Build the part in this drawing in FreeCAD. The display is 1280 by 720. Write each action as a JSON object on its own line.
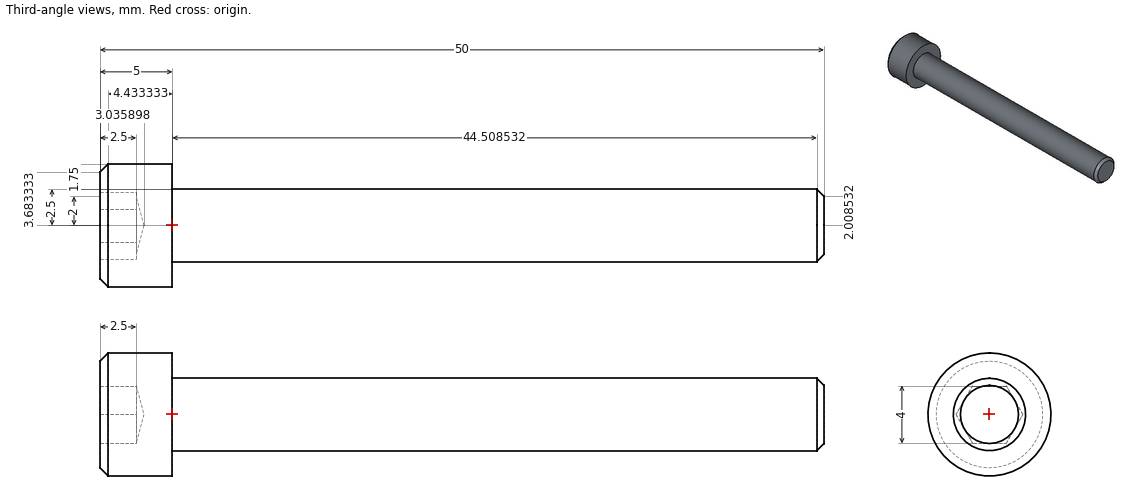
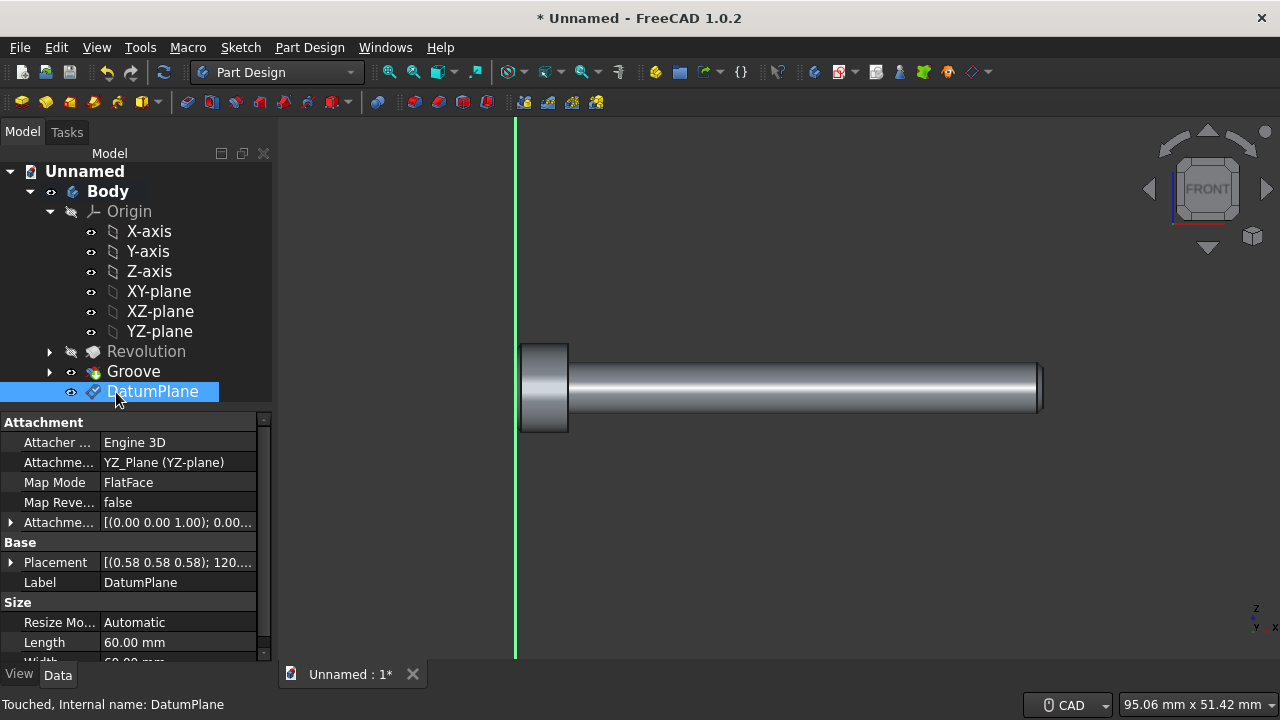
{"action": "left_click", "coordinate": [840, 72]}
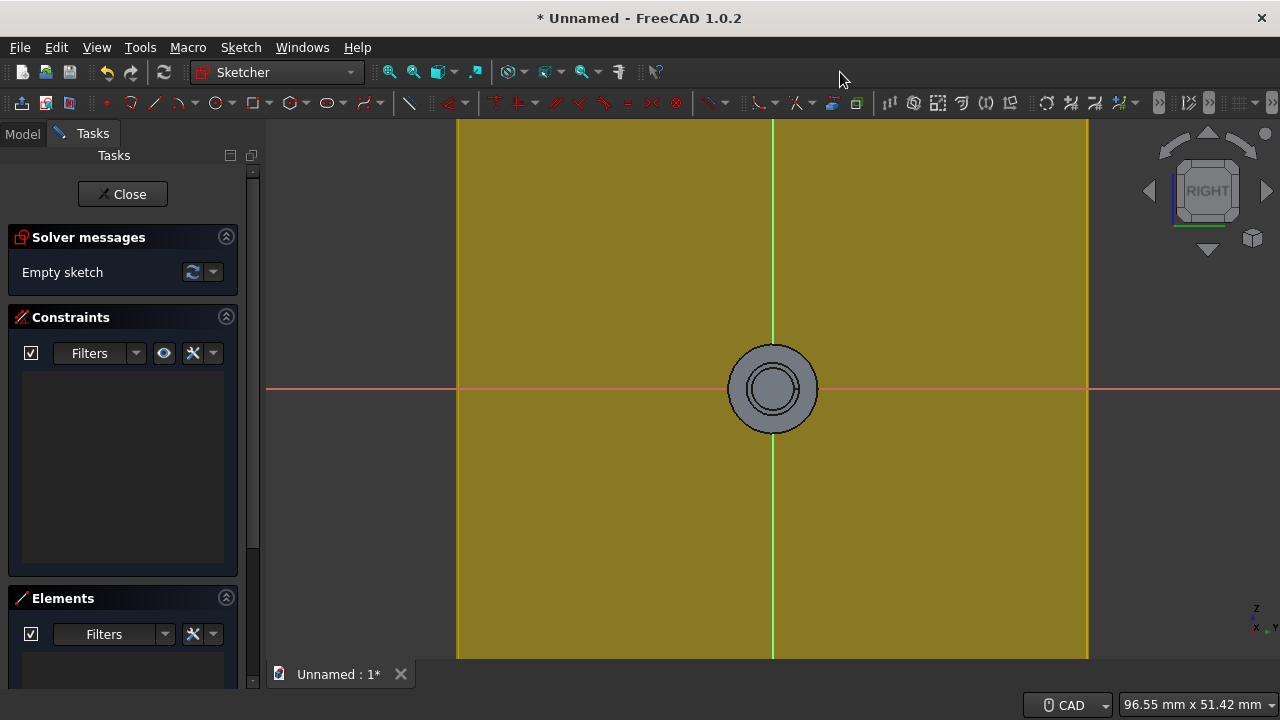
{"action": "key", "text": "q s"}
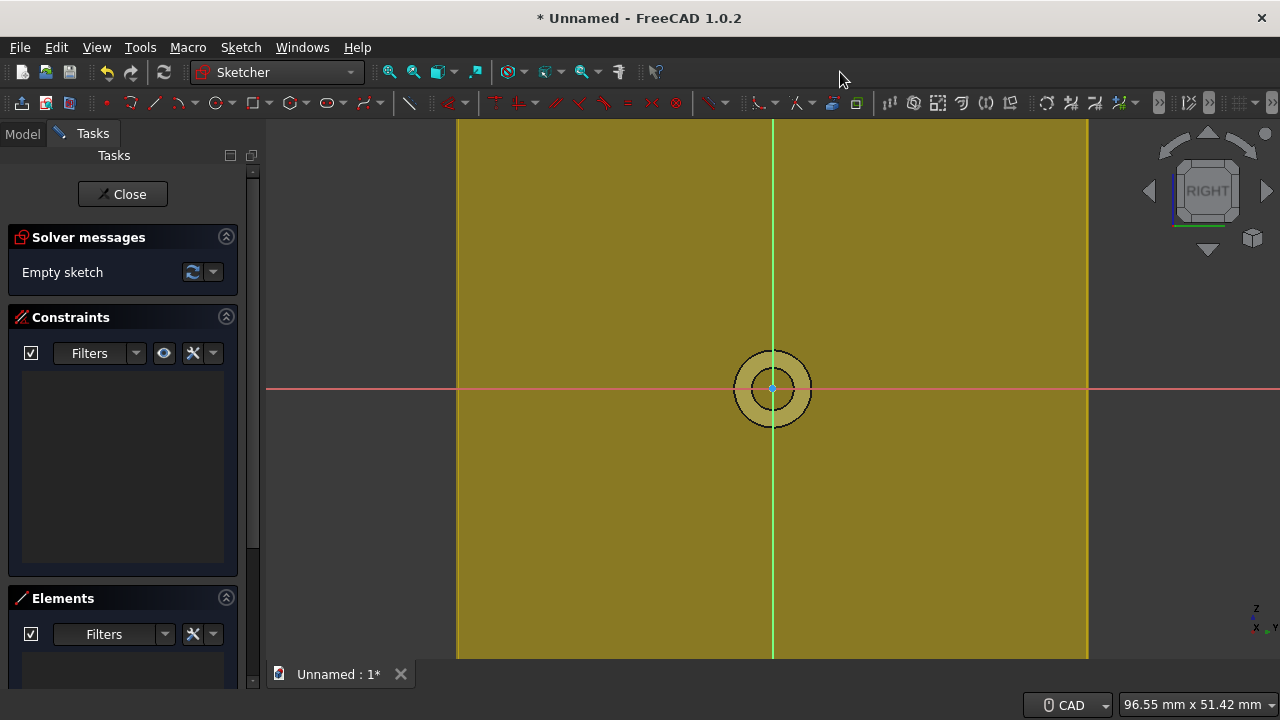
{"action": "scroll", "coordinate": [784, 389], "scroll_direction": "up", "scroll_amount": 10}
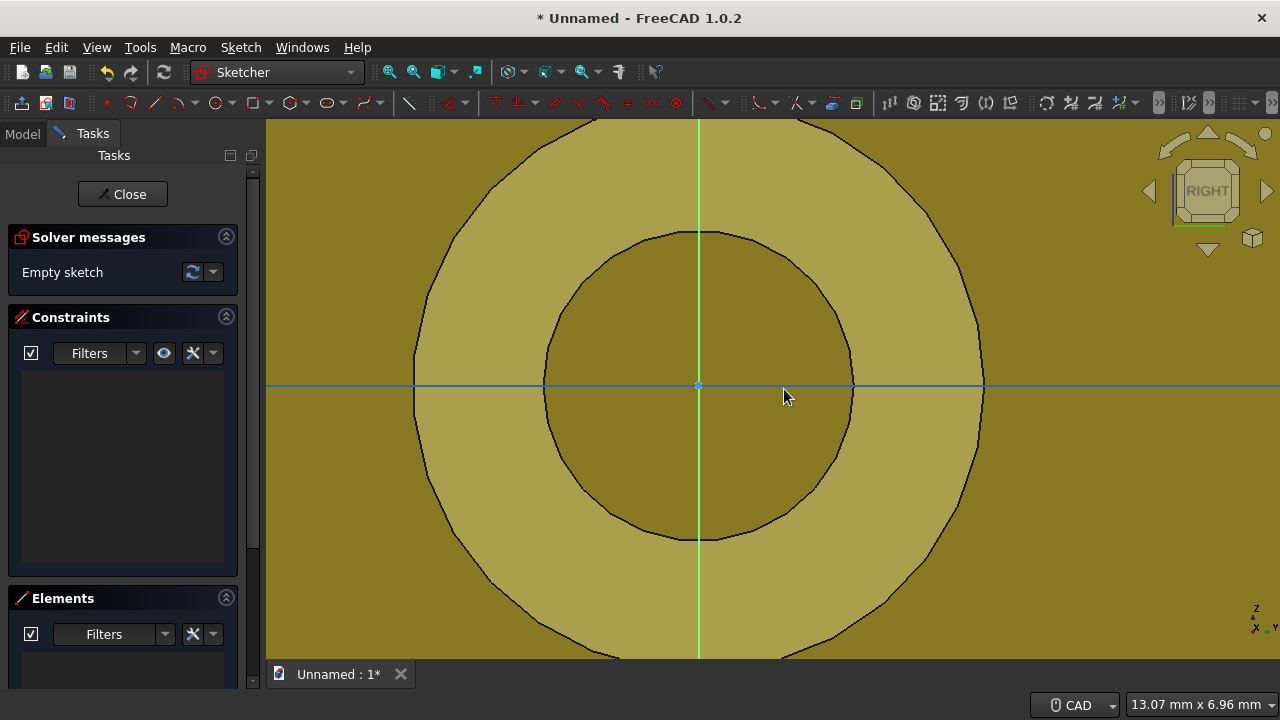
{"action": "left_click", "coordinate": [290, 104]}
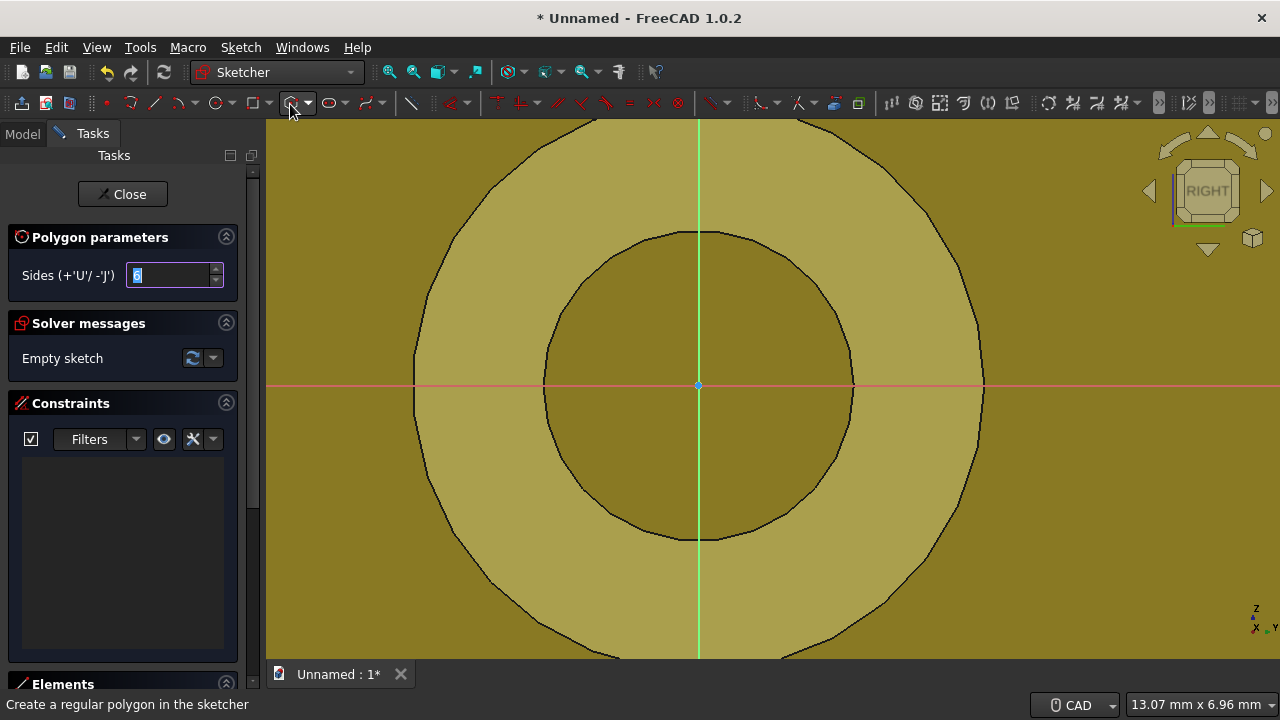
{"action": "left_click", "coordinate": [699, 386]}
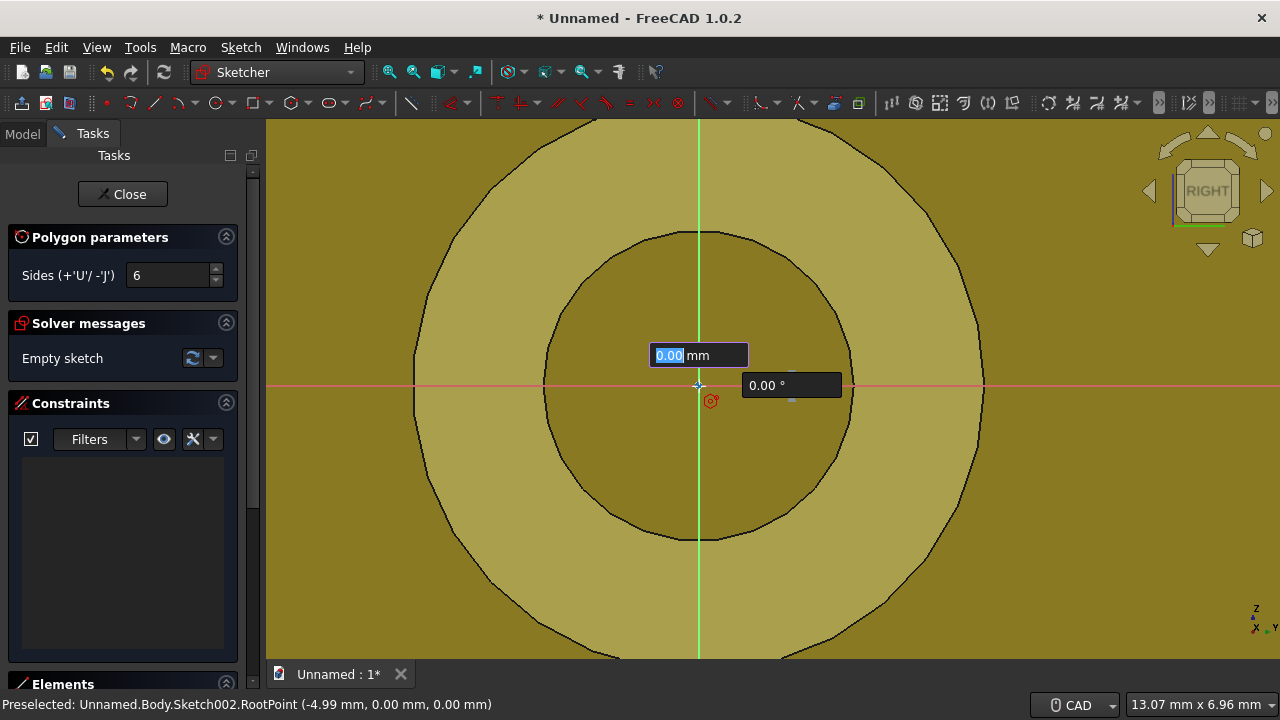
{"action": "left_click", "coordinate": [519, 386]}
{"action": "right_click", "coordinate": [519, 386]}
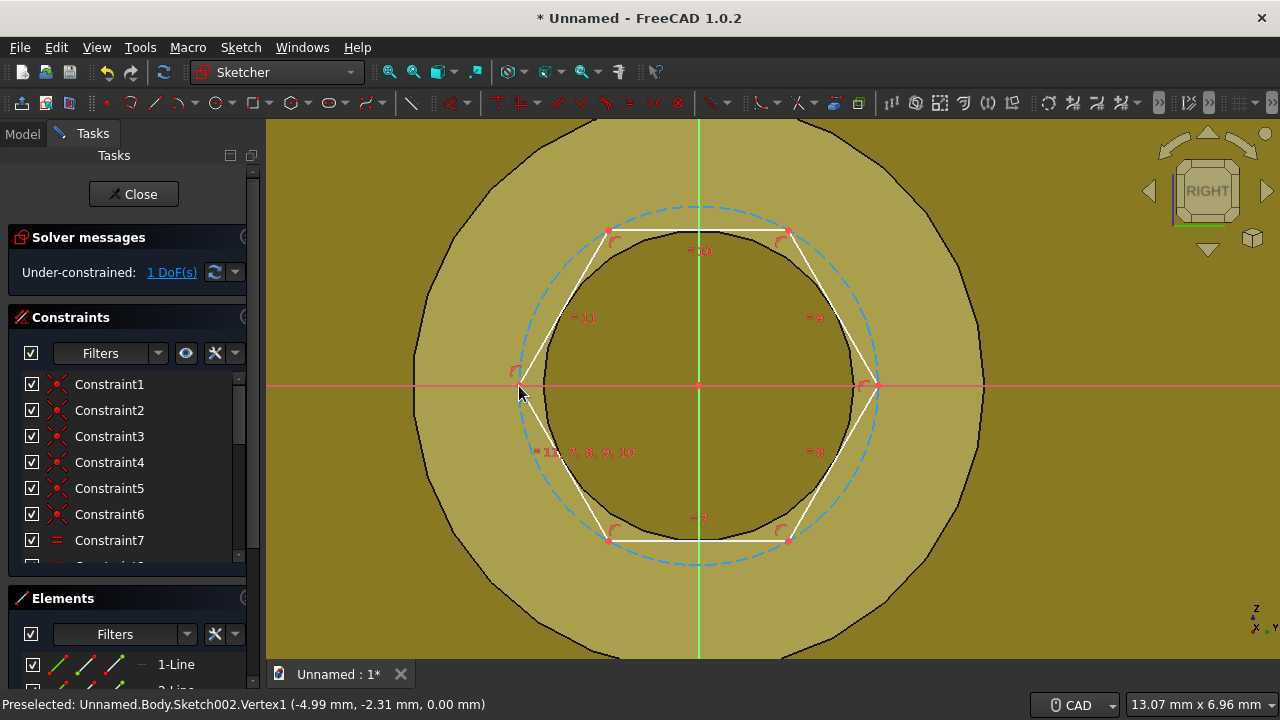
{"action": "key", "text": "d"}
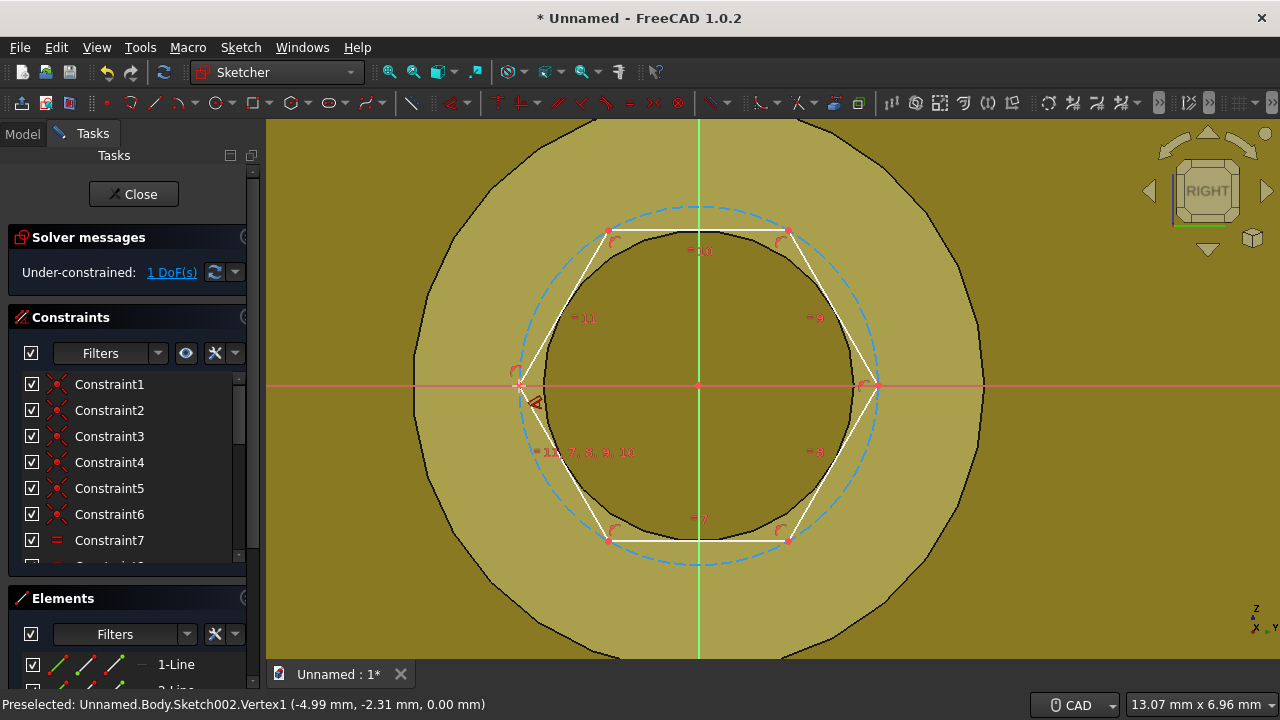
{"action": "left_click", "coordinate": [609, 541]}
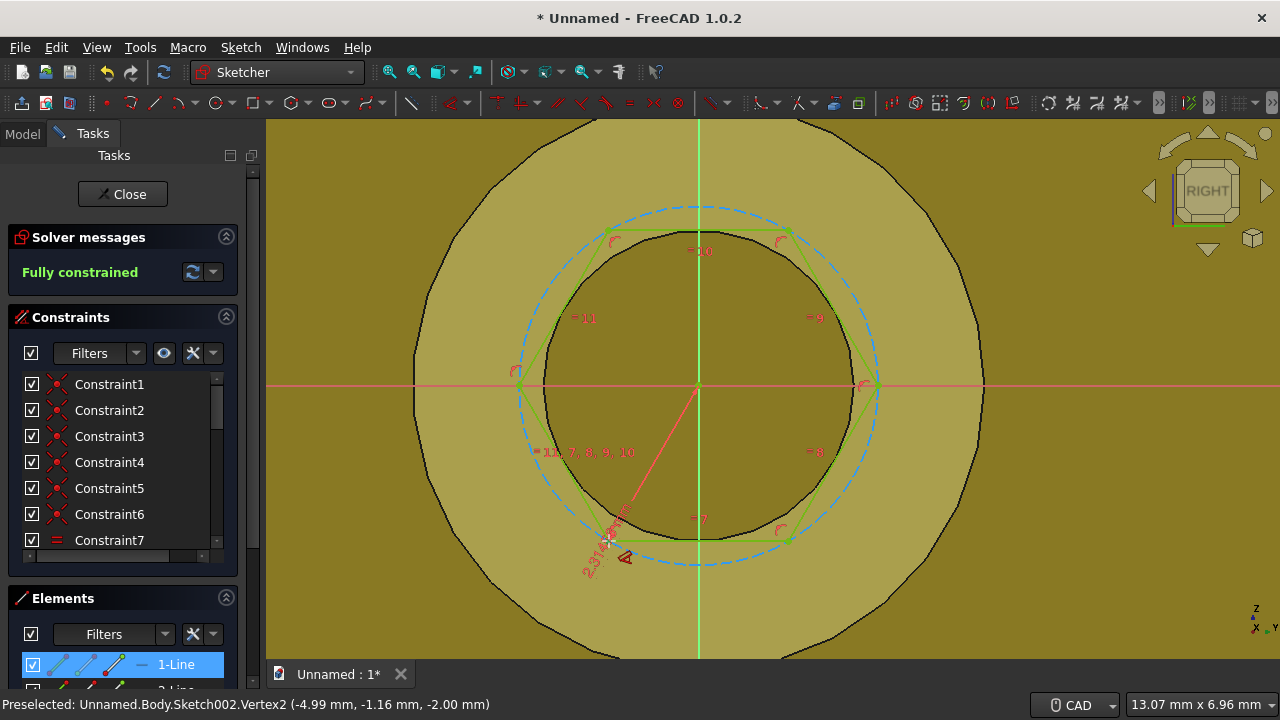
{"action": "left_click", "coordinate": [788, 230]}
{"action": "left_click", "coordinate": [870, 277]}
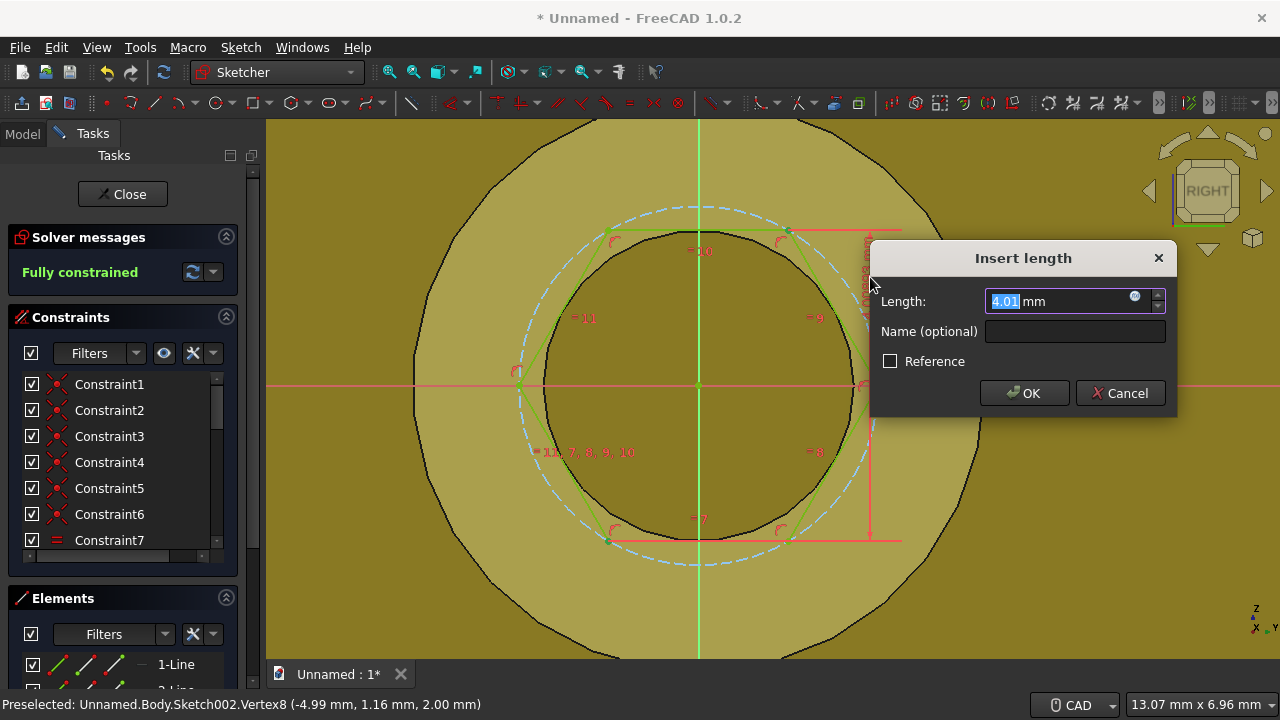
{"action": "type", "text": "4"}
{"action": "key", "text": "Return"}
{"action": "key", "text": "Escape"}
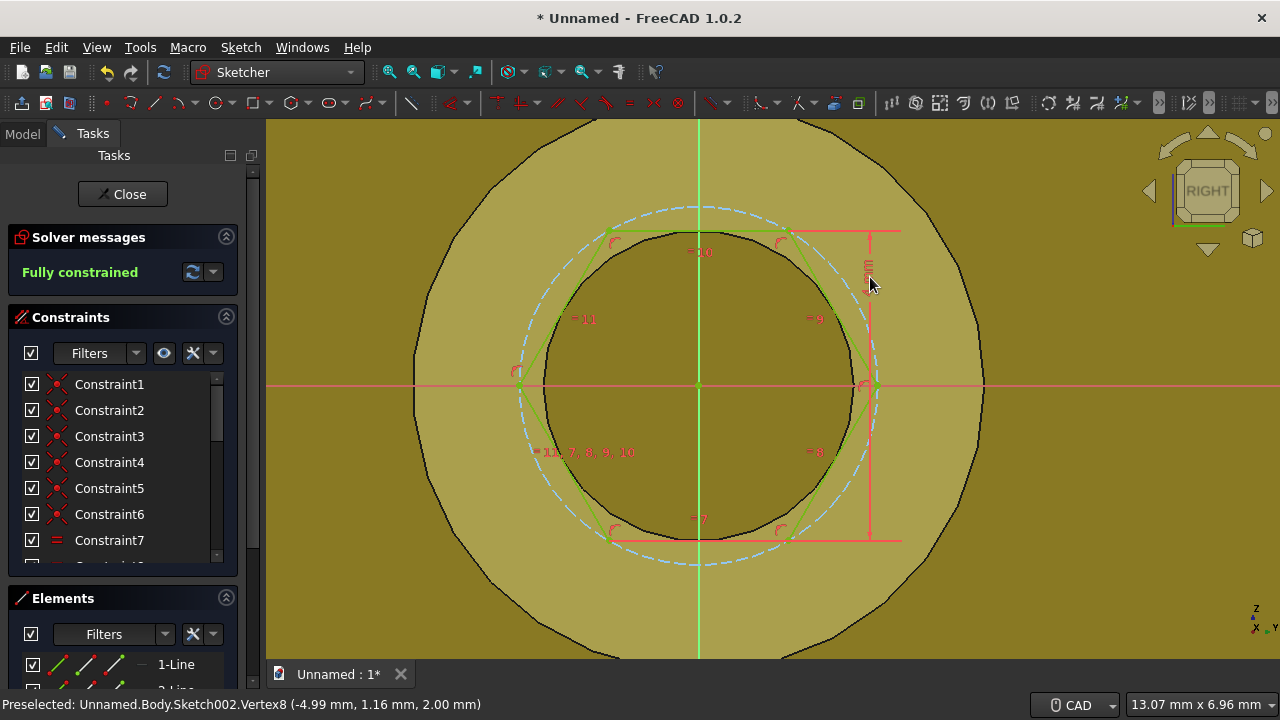
{"action": "left_click", "coordinate": [123, 194]}